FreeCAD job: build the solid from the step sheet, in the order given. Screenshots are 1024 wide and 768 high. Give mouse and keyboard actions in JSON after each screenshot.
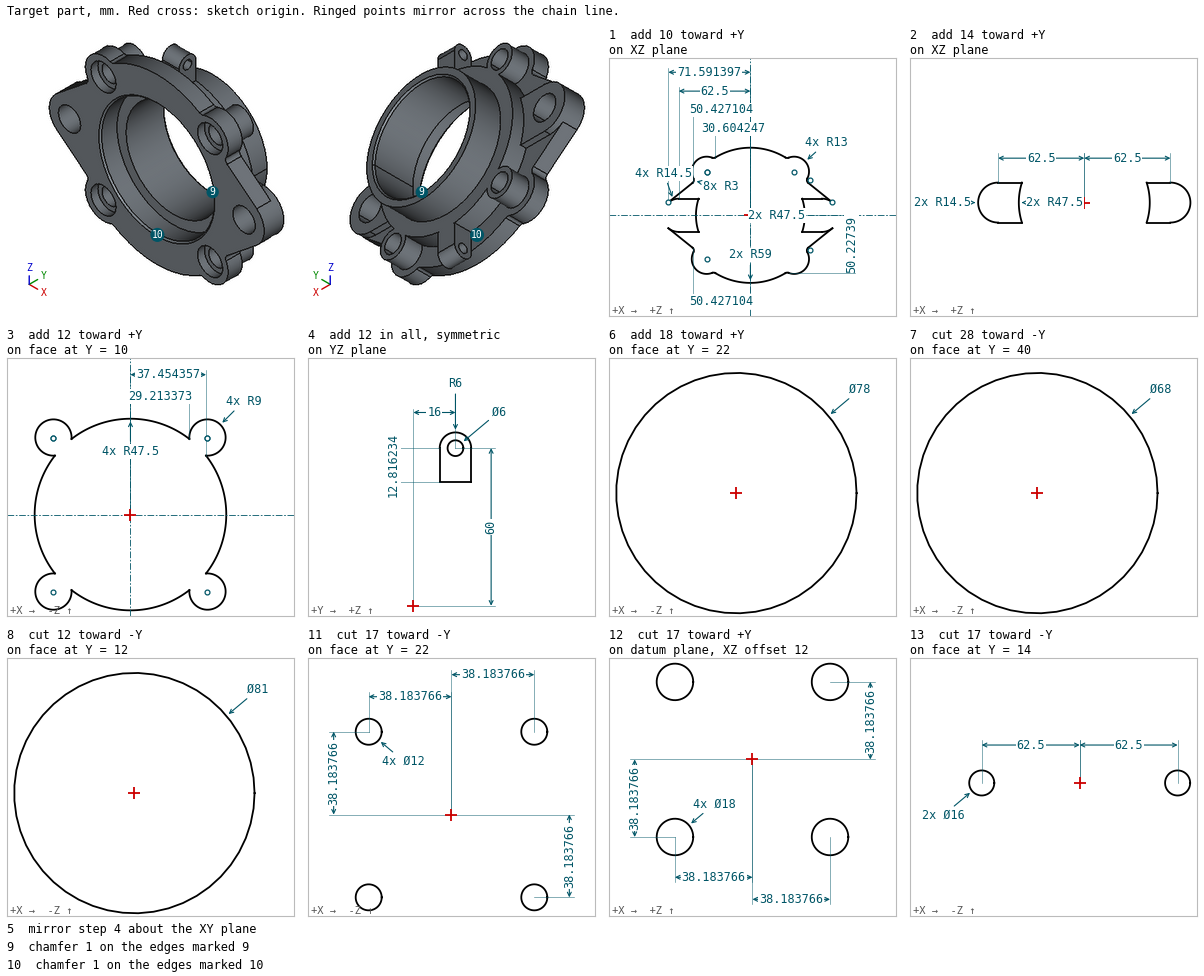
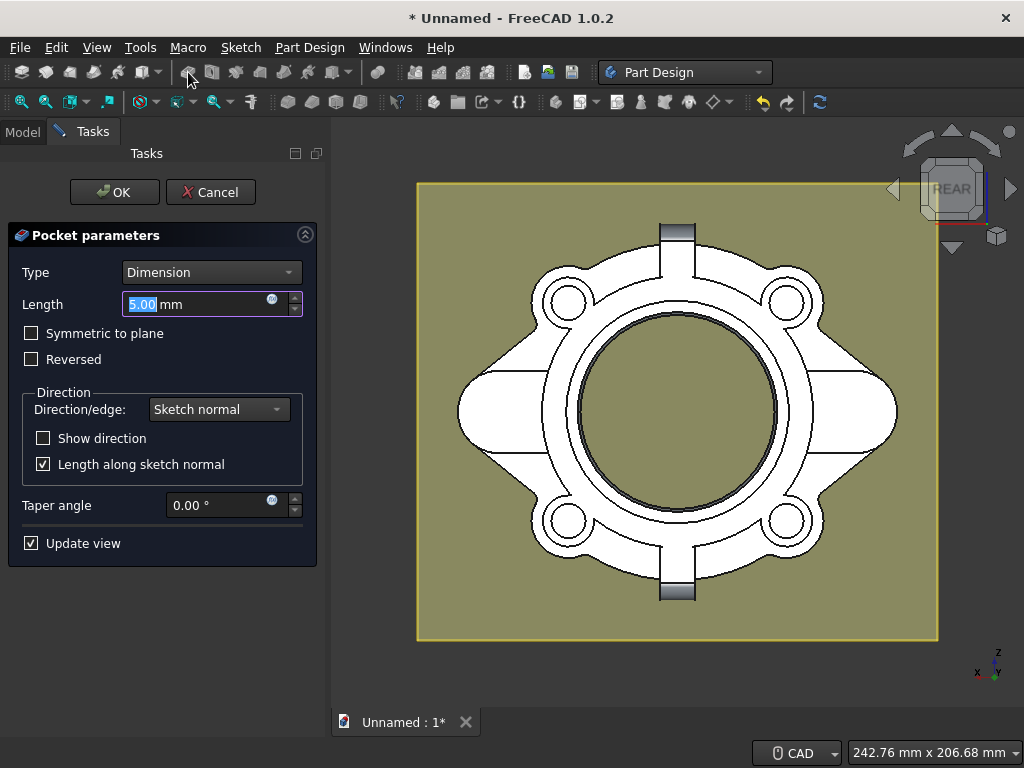
{"action": "type", "text": "17"}
{"action": "key", "text": "Tab"}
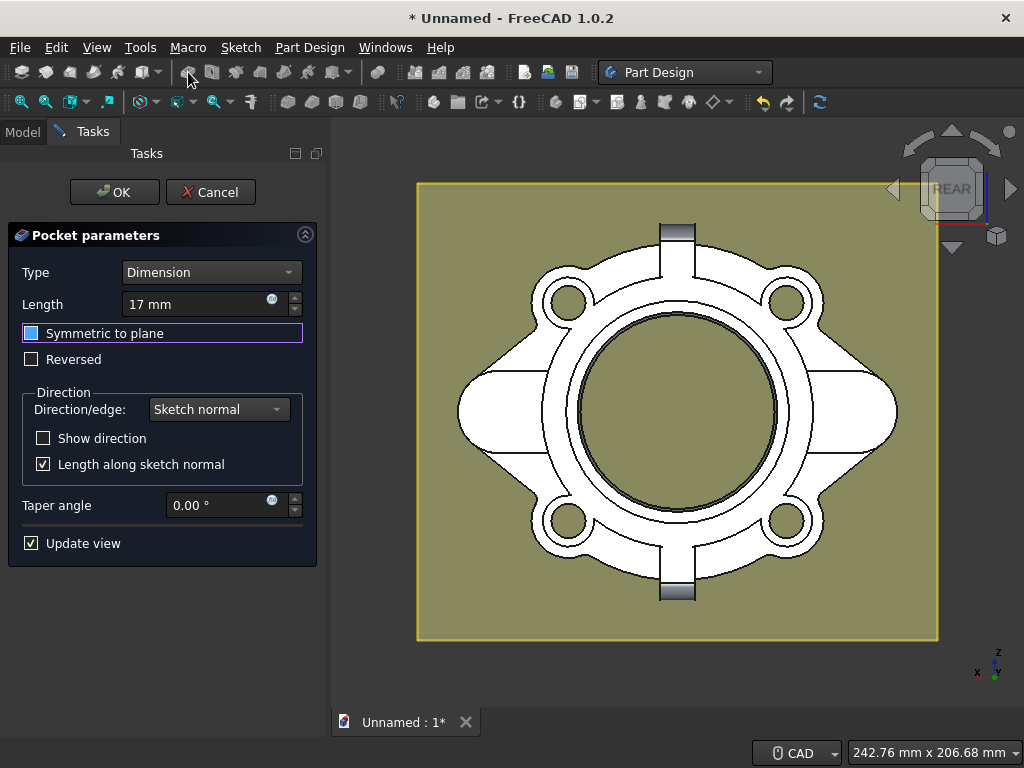
{"action": "left_click", "coordinate": [115, 192]}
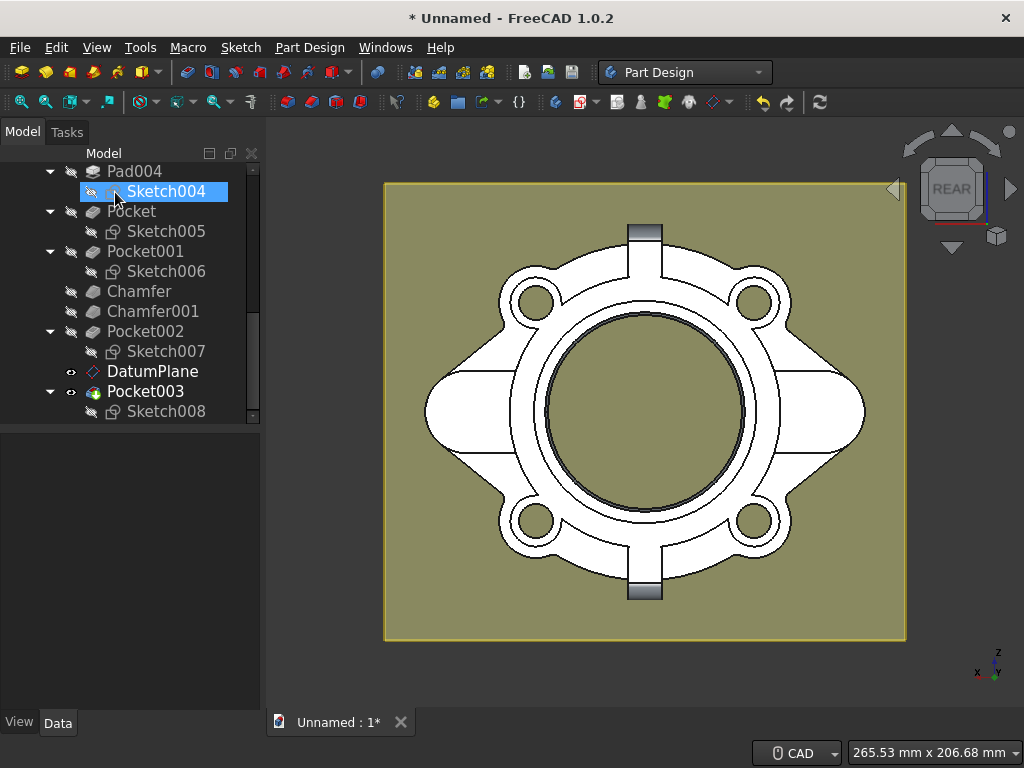
{"action": "left_click", "coordinate": [116, 372]}
{"action": "key", "text": "space"}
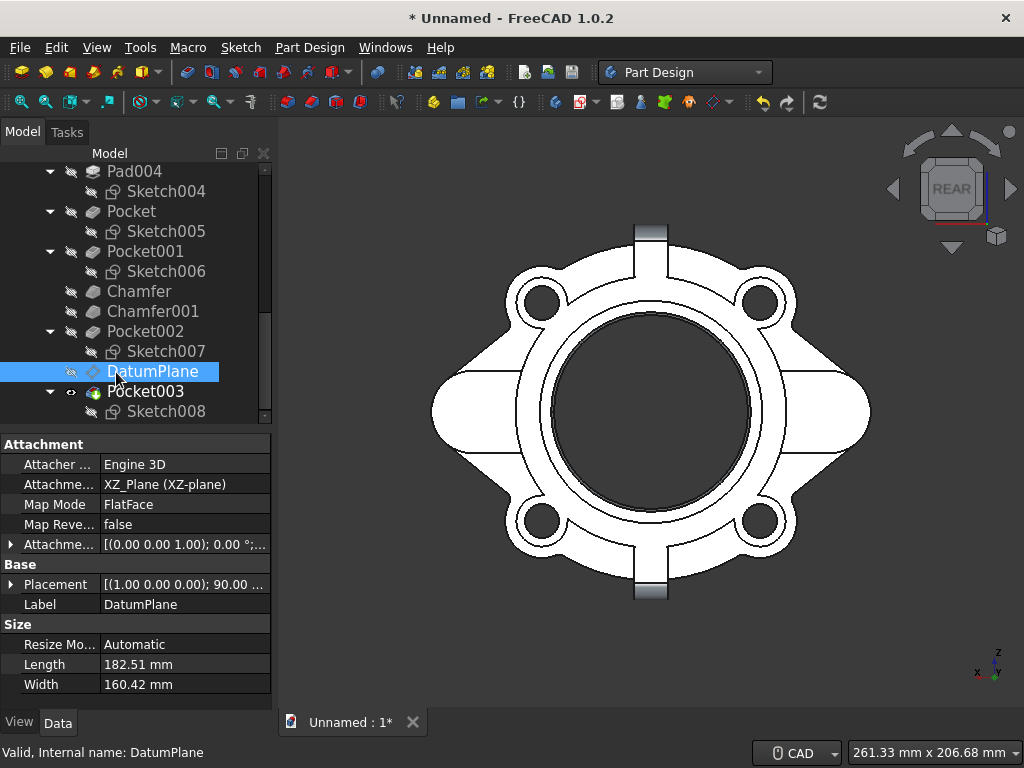
{"action": "left_click", "coordinate": [477, 411]}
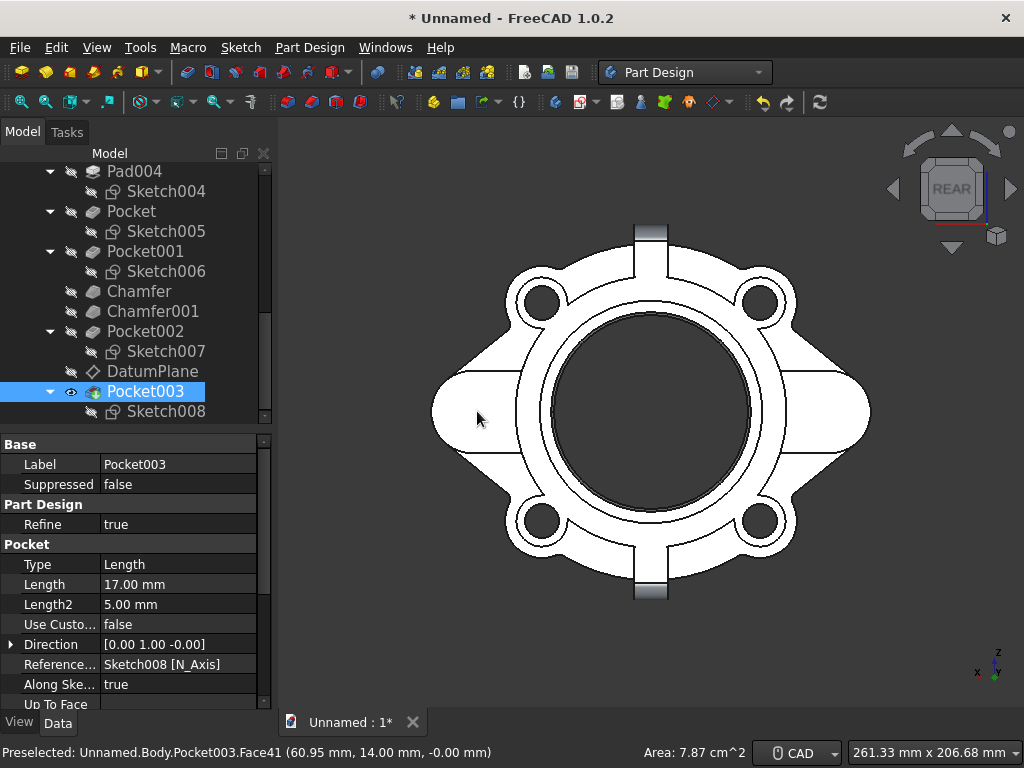
{"action": "left_click", "coordinate": [580, 102]}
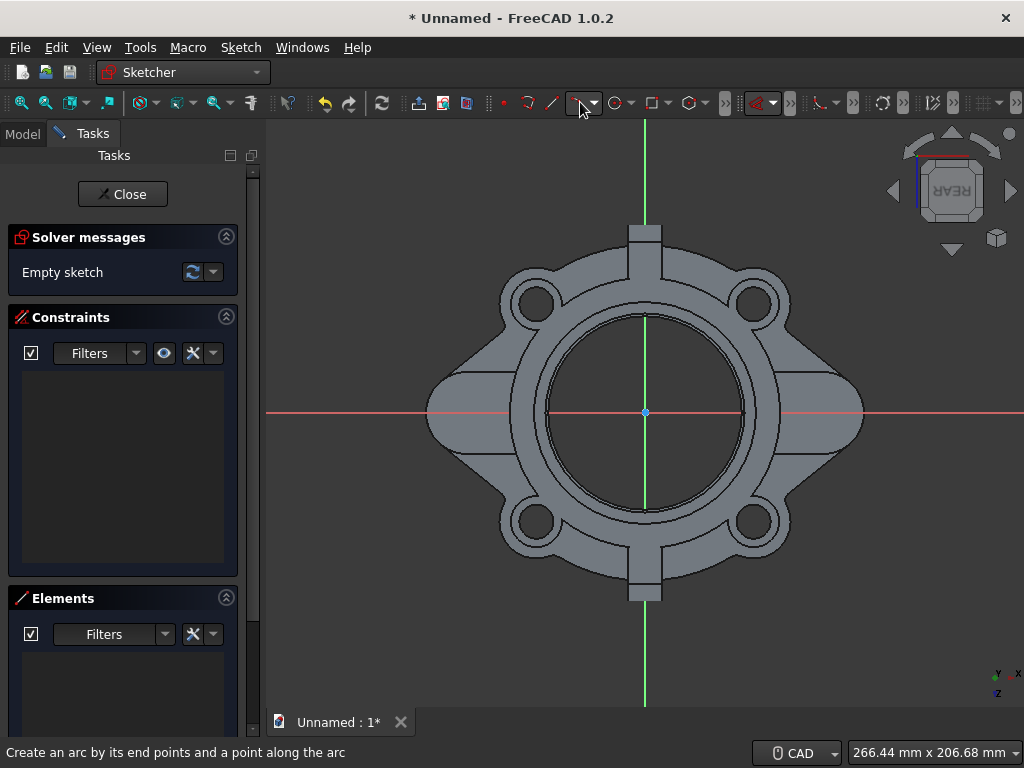
{"action": "key", "text": "q s"}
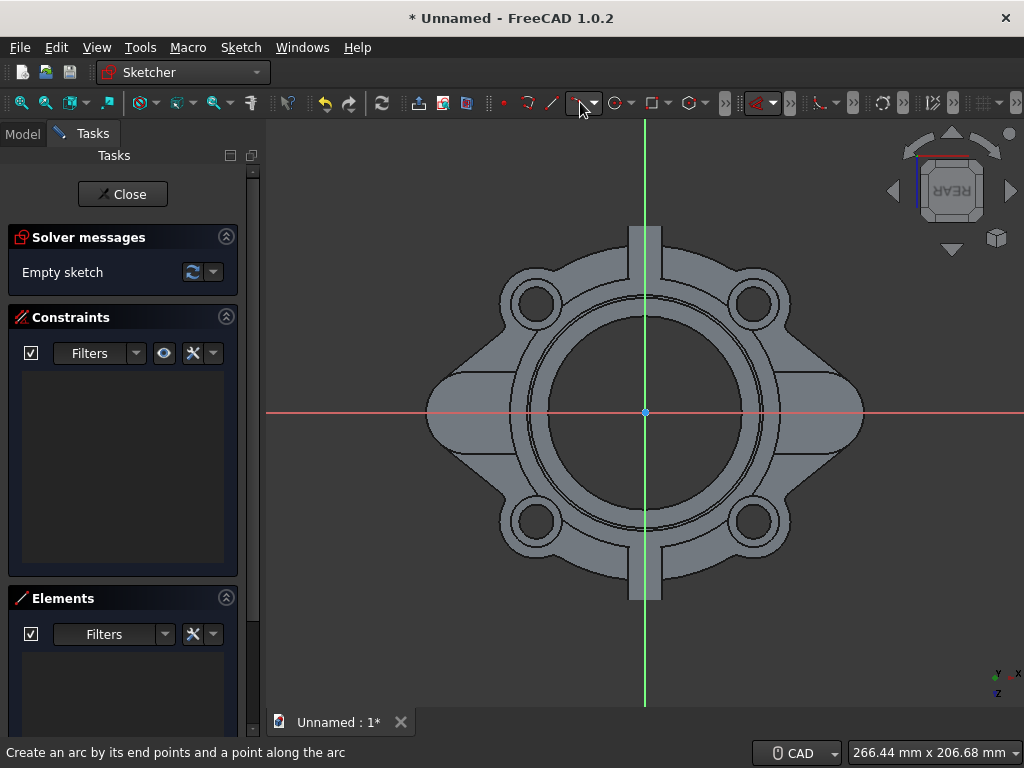
{"action": "scroll", "coordinate": [294, 413], "scroll_direction": "down", "scroll_amount": 1}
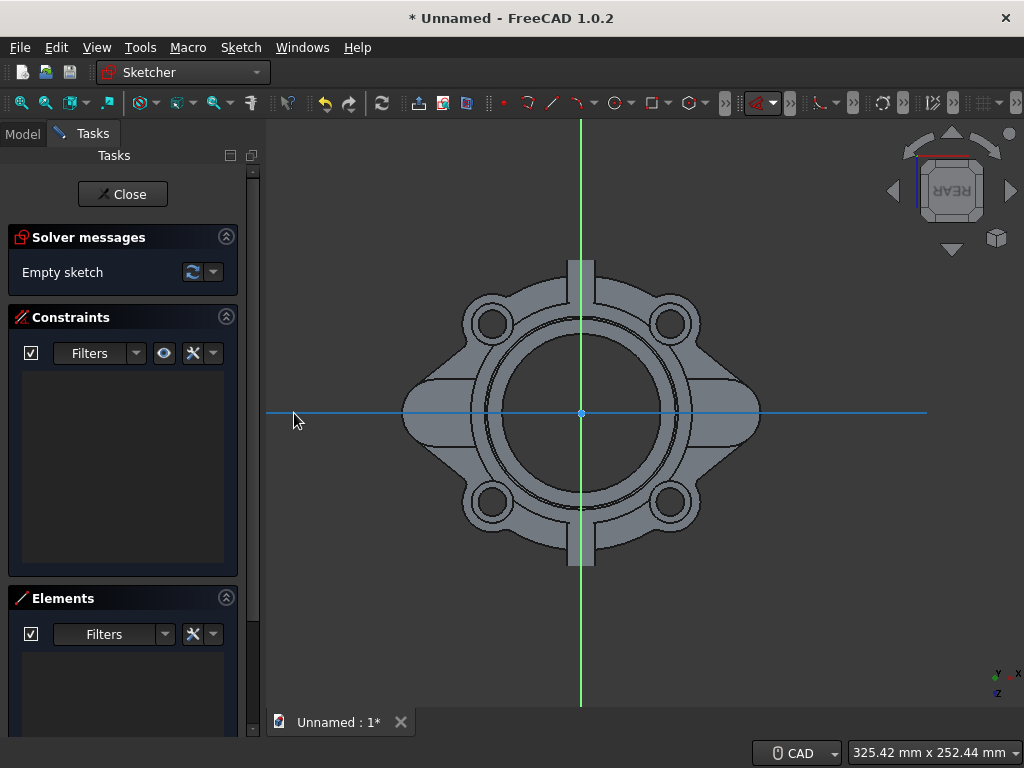
{"action": "key", "text": "g c"}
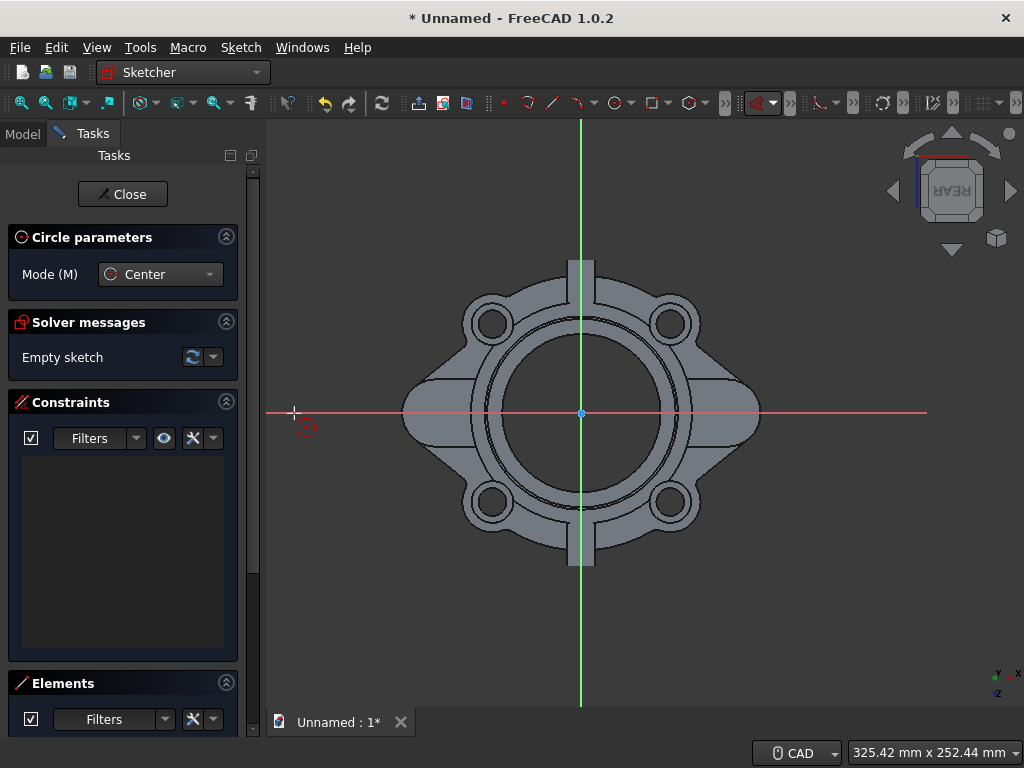
{"action": "left_click", "coordinate": [436, 413]}
{"action": "left_click", "coordinate": [442, 396]}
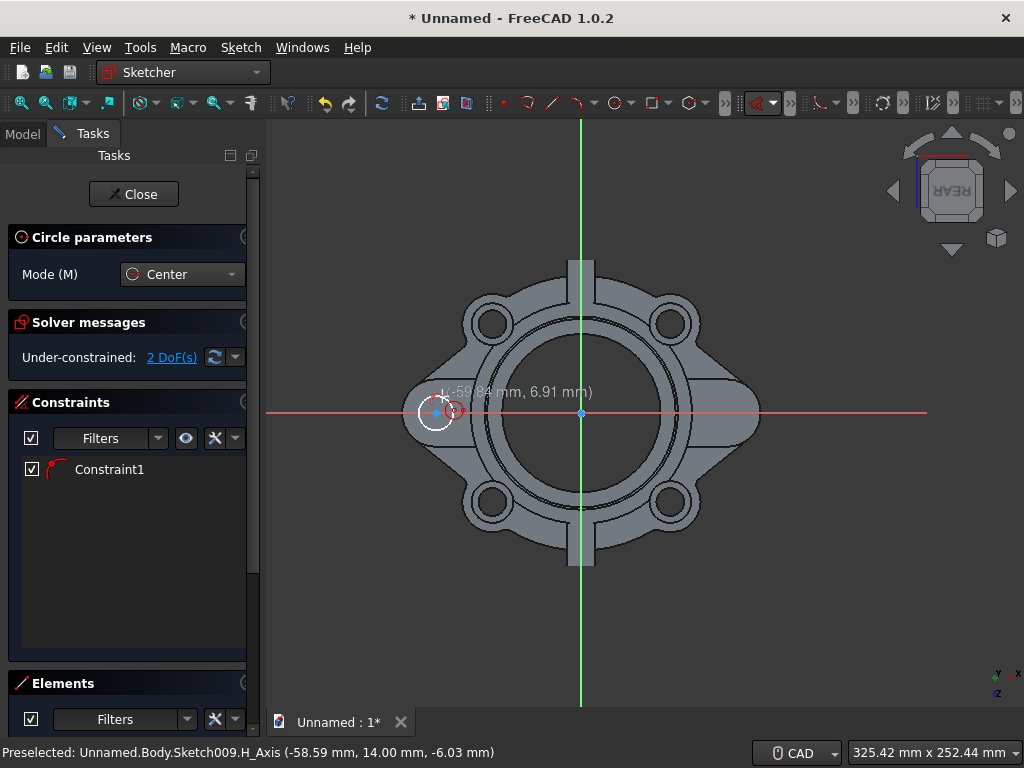
{"action": "left_click", "coordinate": [727, 413]}
{"action": "left_click", "coordinate": [733, 396]}
{"action": "key", "text": "Escape"}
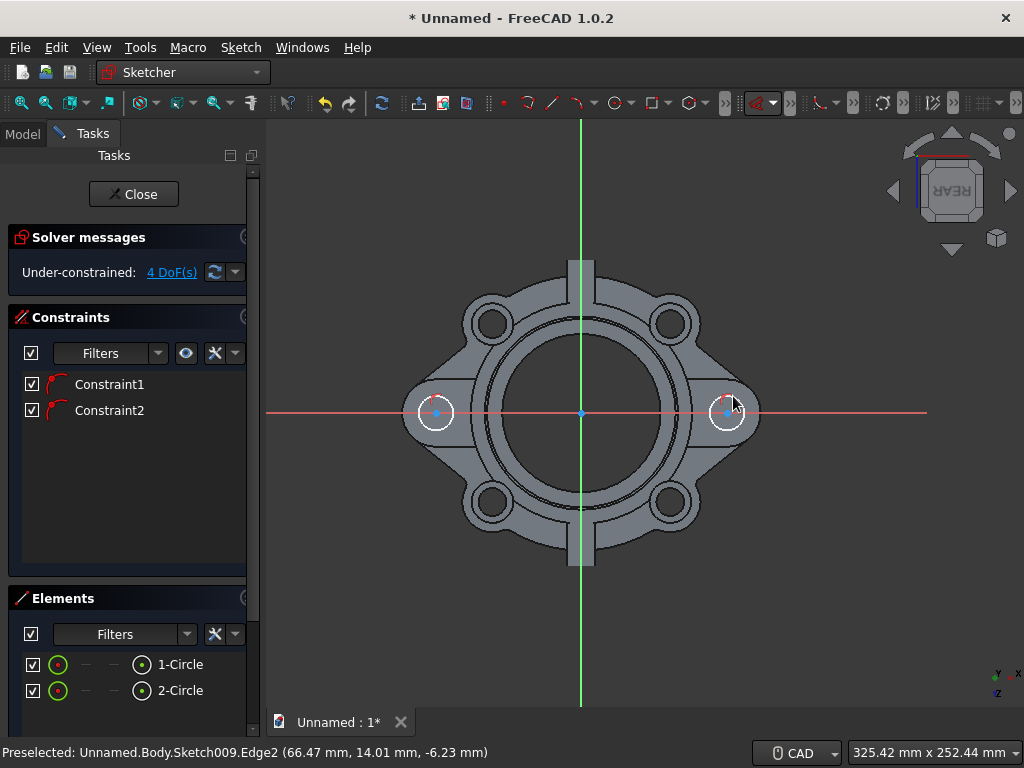
{"action": "left_click", "coordinate": [448, 401]}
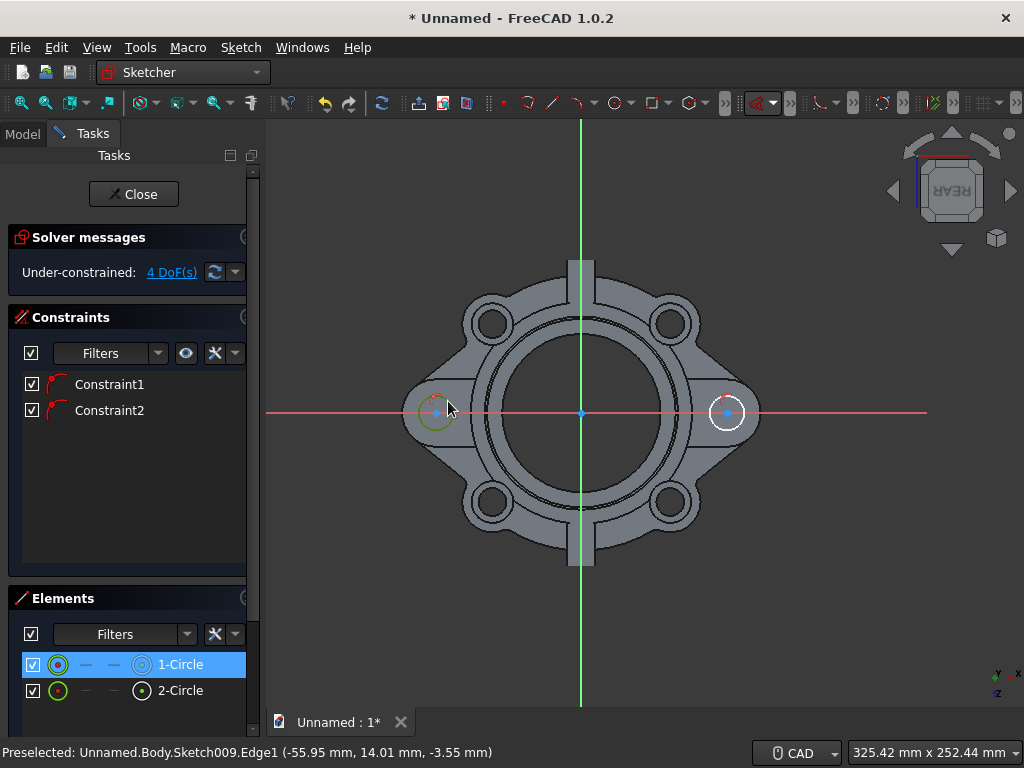
{"action": "left_click", "coordinate": [739, 401]}